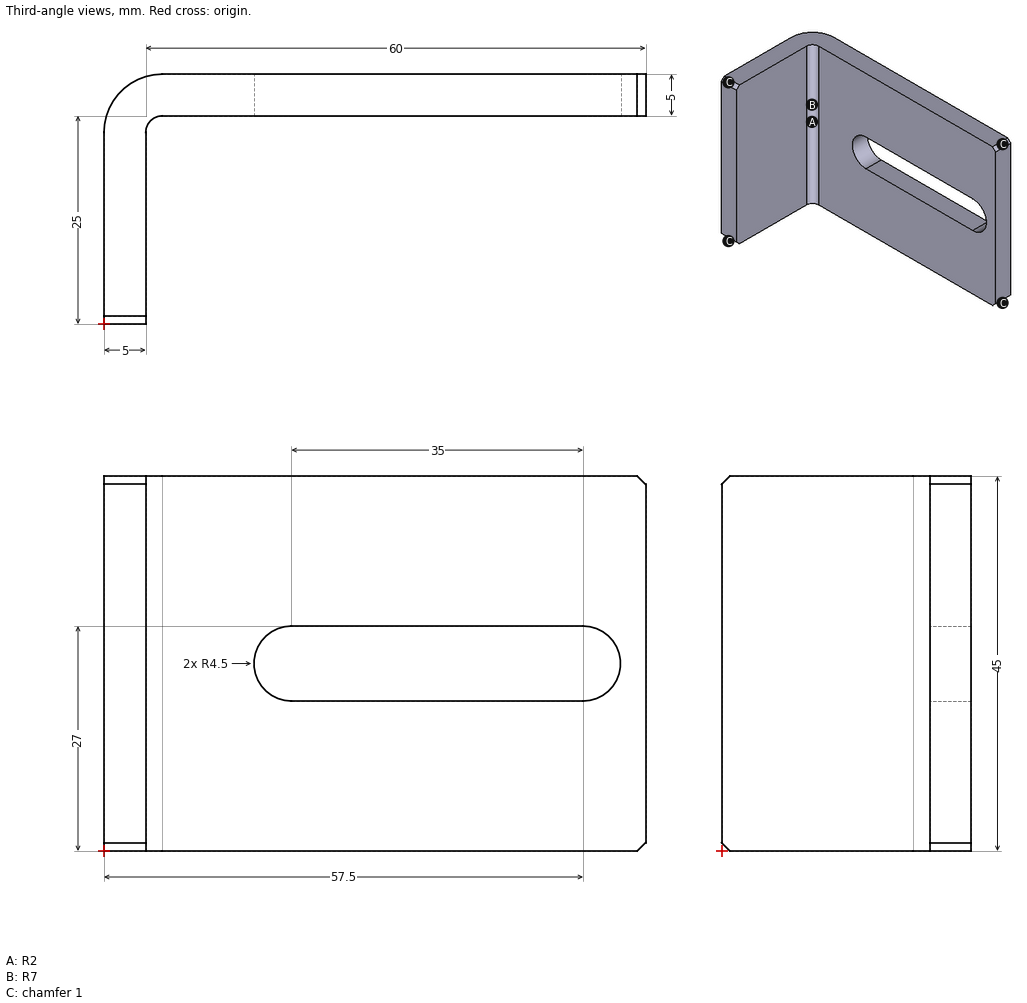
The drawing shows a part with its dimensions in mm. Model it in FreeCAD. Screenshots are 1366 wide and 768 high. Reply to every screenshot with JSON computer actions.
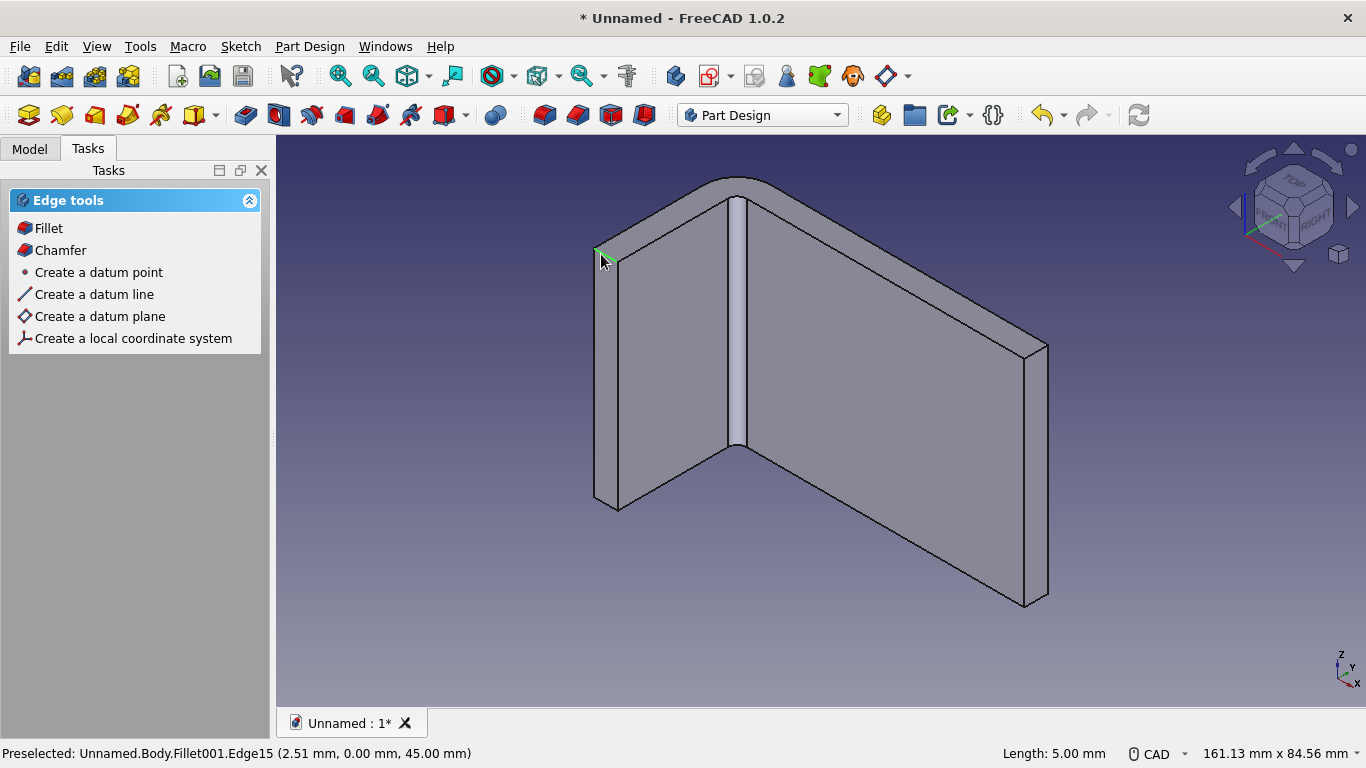
{"action": "left_click", "coordinate": [1036, 351], "text": "ctrl"}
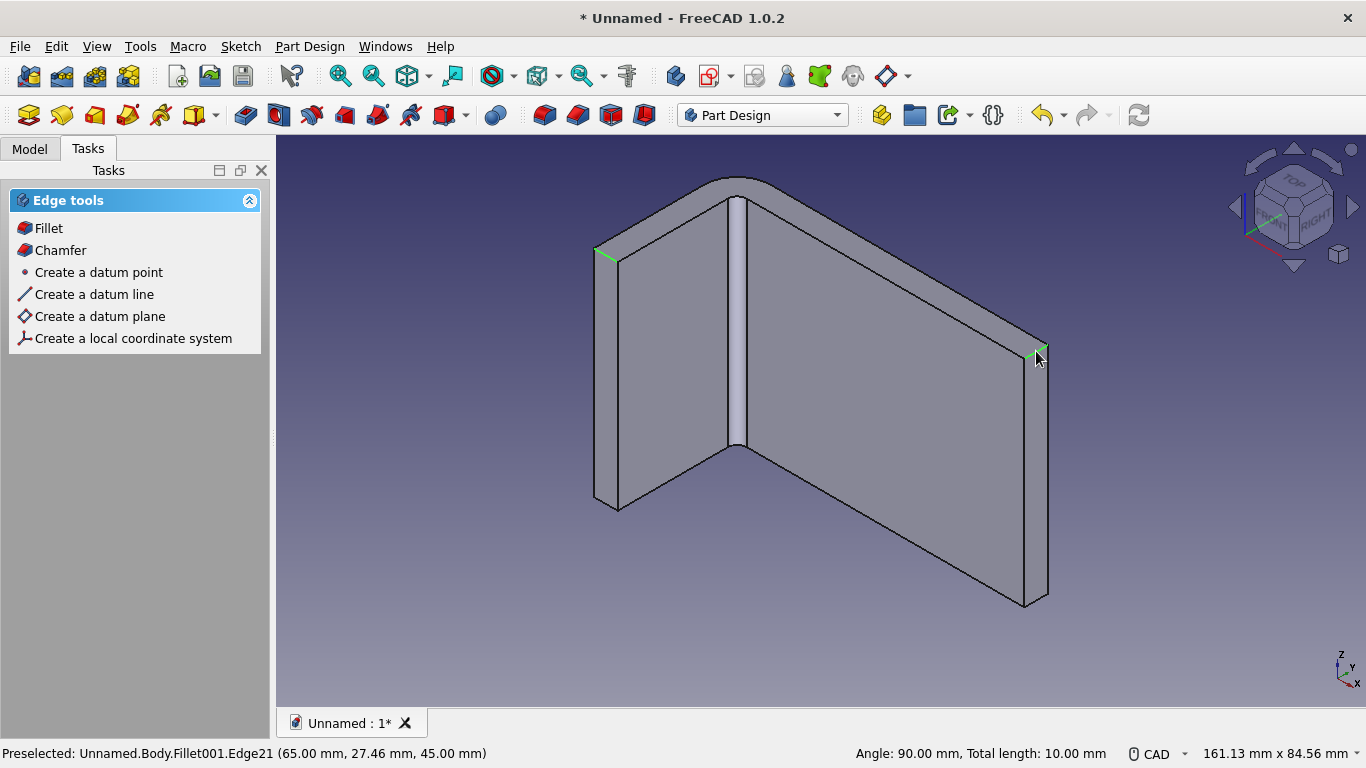
{"action": "key", "text": "2"}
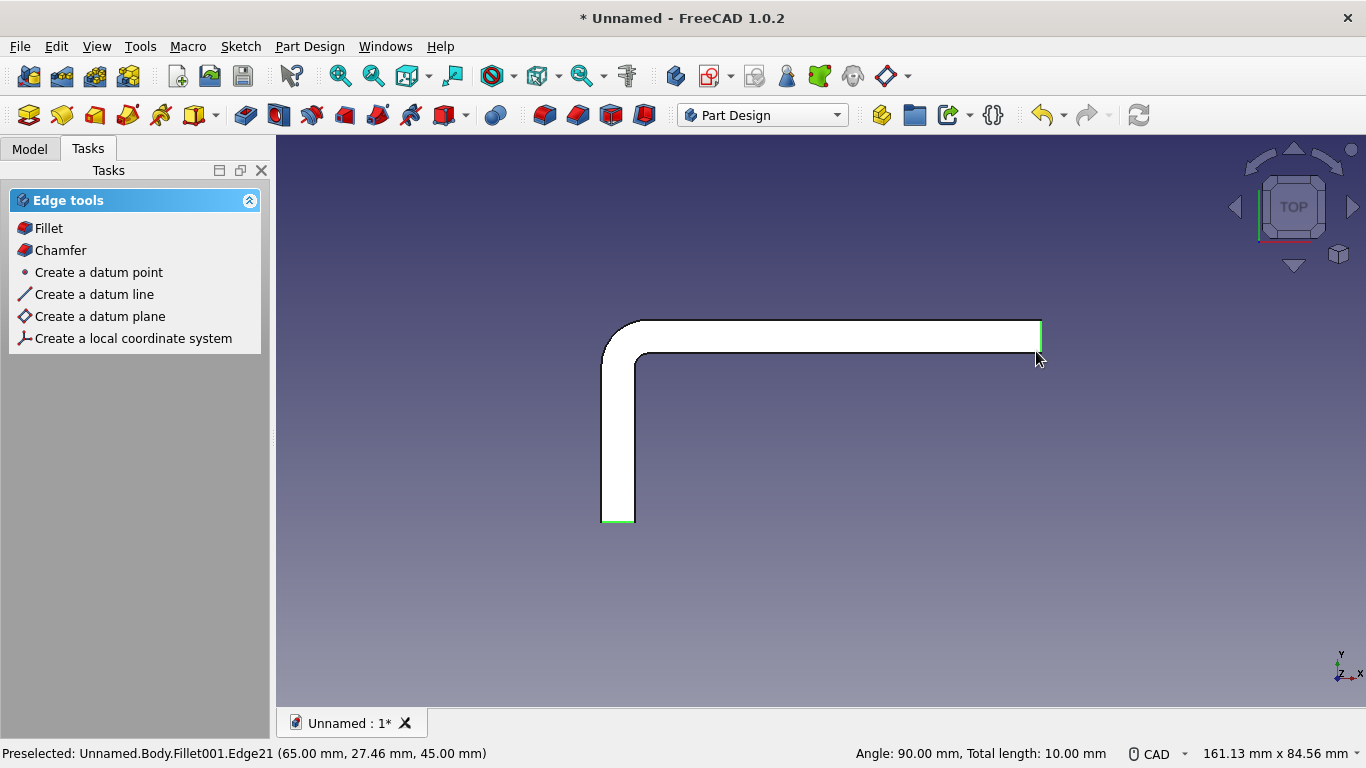
{"action": "left_click", "coordinate": [341, 76]}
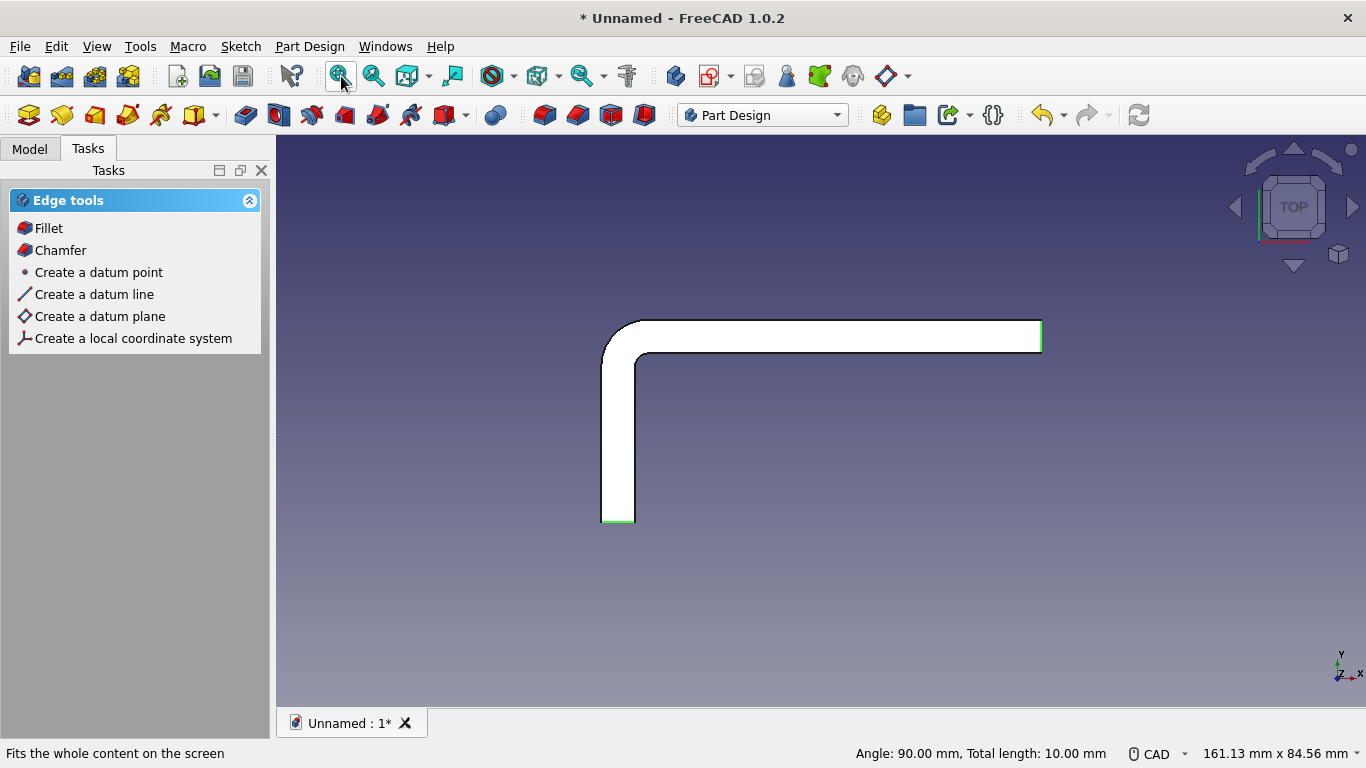
{"action": "key", "text": "1"}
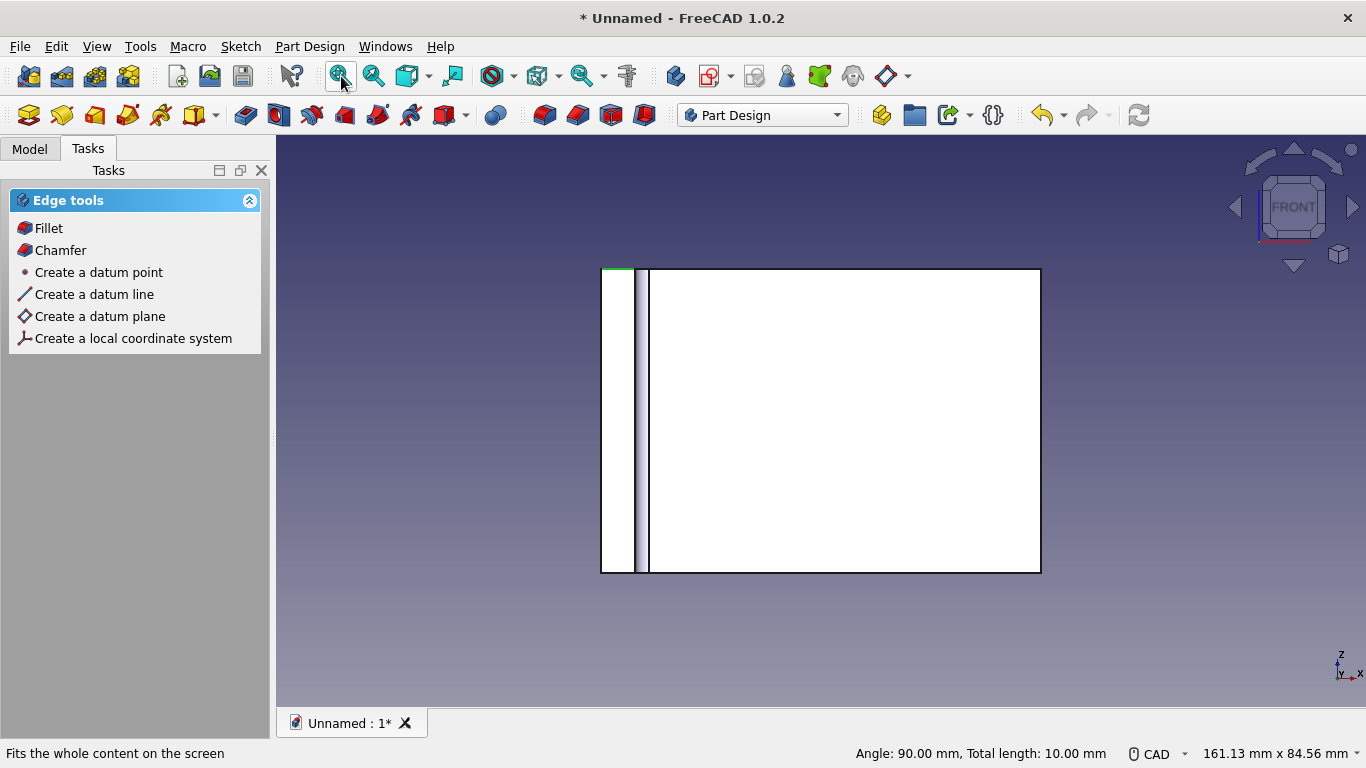
{"action": "left_click", "coordinate": [618, 572], "text": "ctrl"}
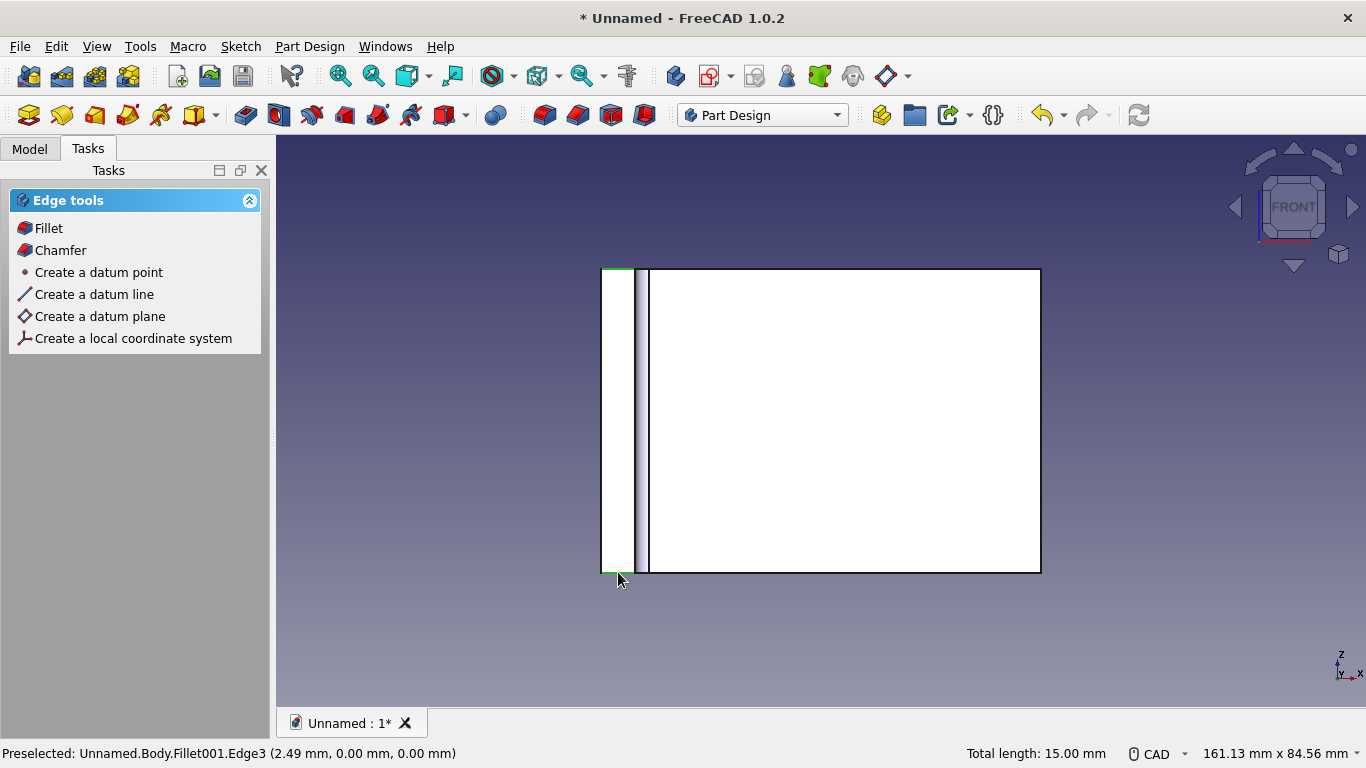
{"action": "key", "text": "3"}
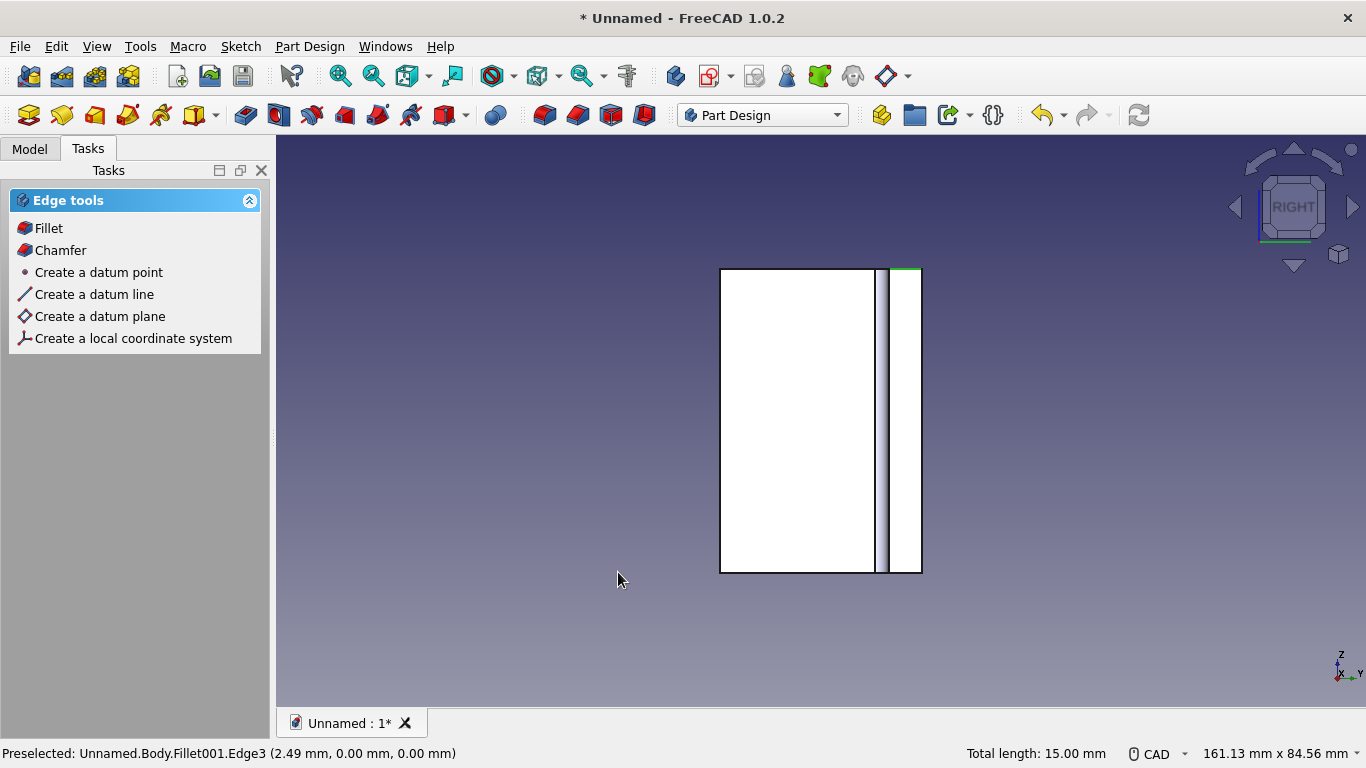
{"action": "left_click", "coordinate": [906, 572], "text": "ctrl"}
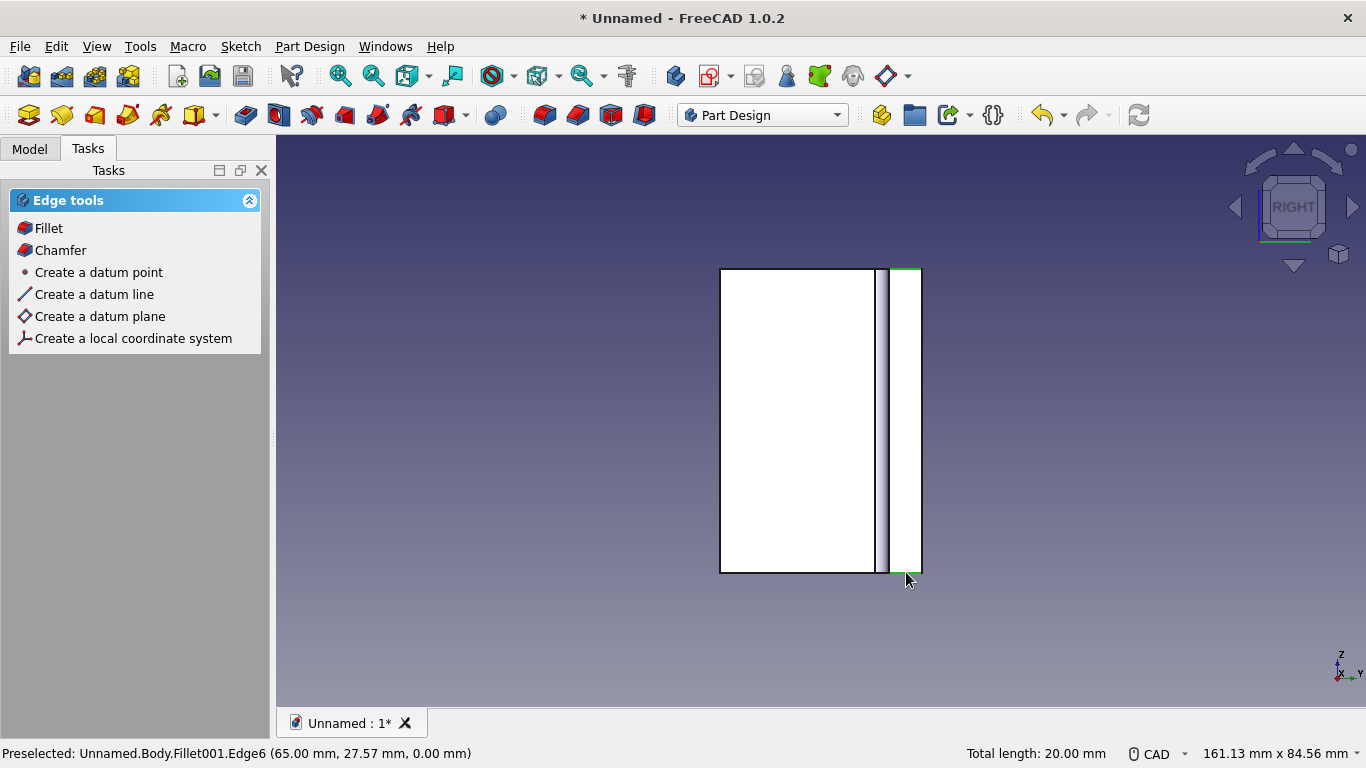
{"action": "left_click", "coordinate": [578, 116]}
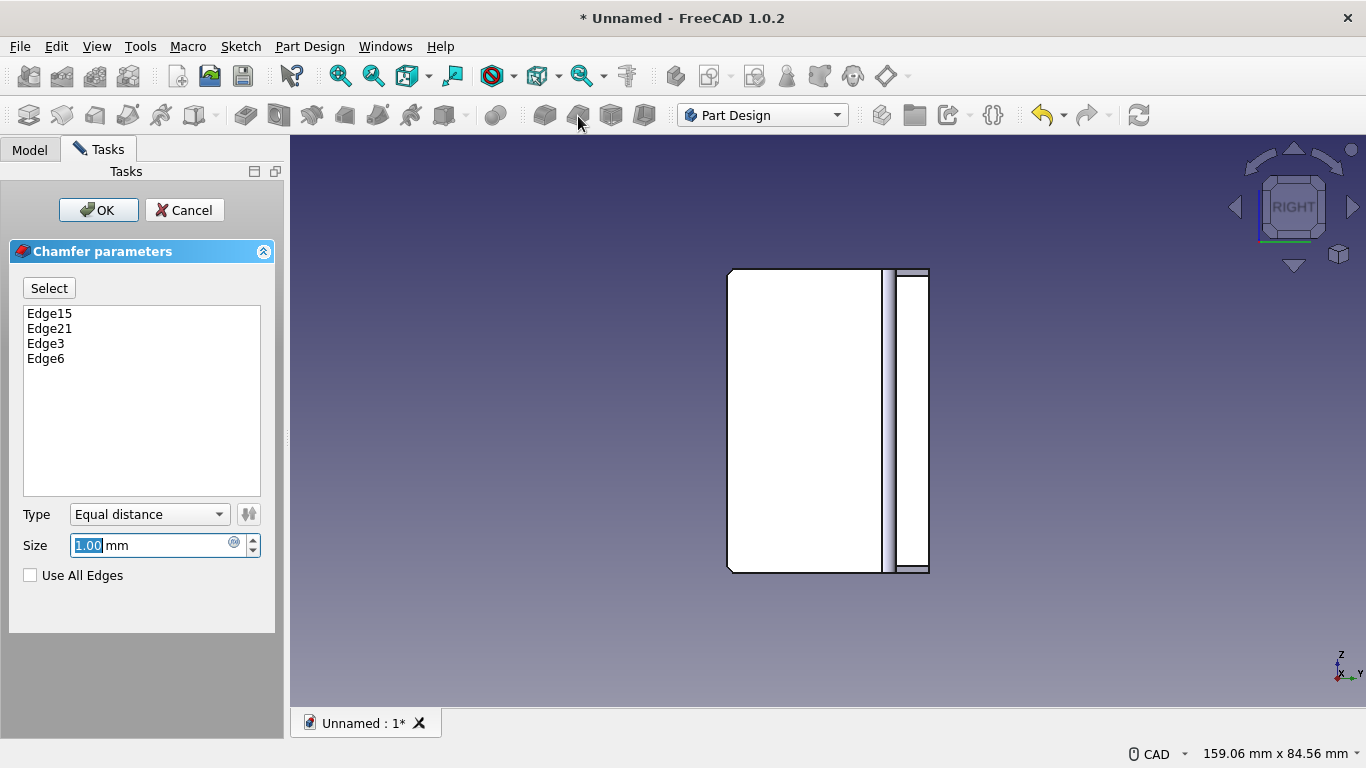
{"action": "type", "text": "1"}
{"action": "key", "text": "Tab"}